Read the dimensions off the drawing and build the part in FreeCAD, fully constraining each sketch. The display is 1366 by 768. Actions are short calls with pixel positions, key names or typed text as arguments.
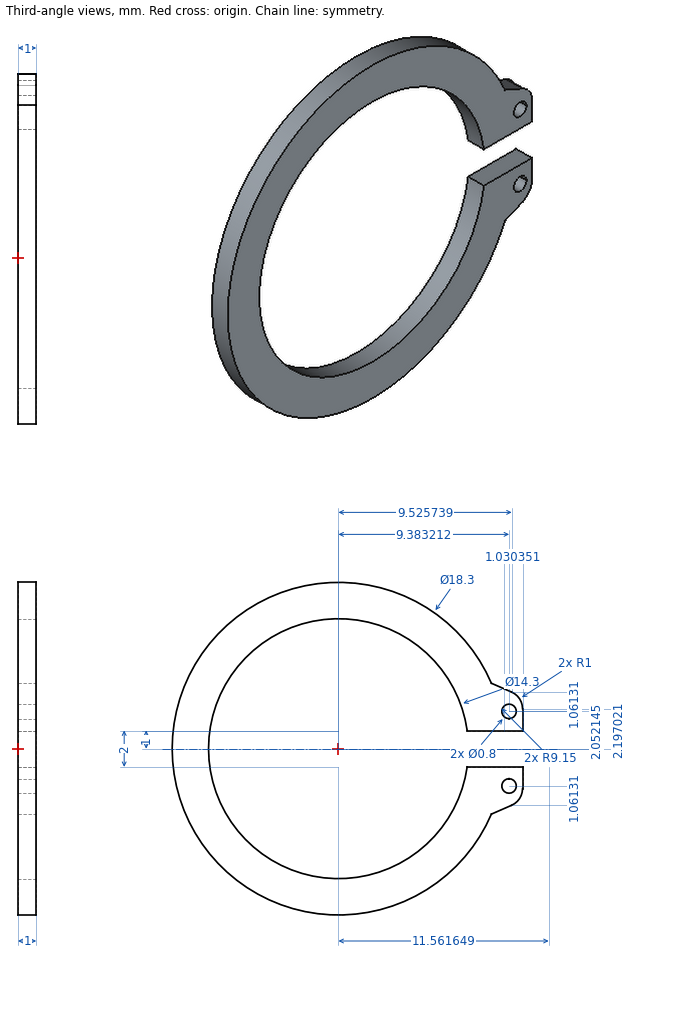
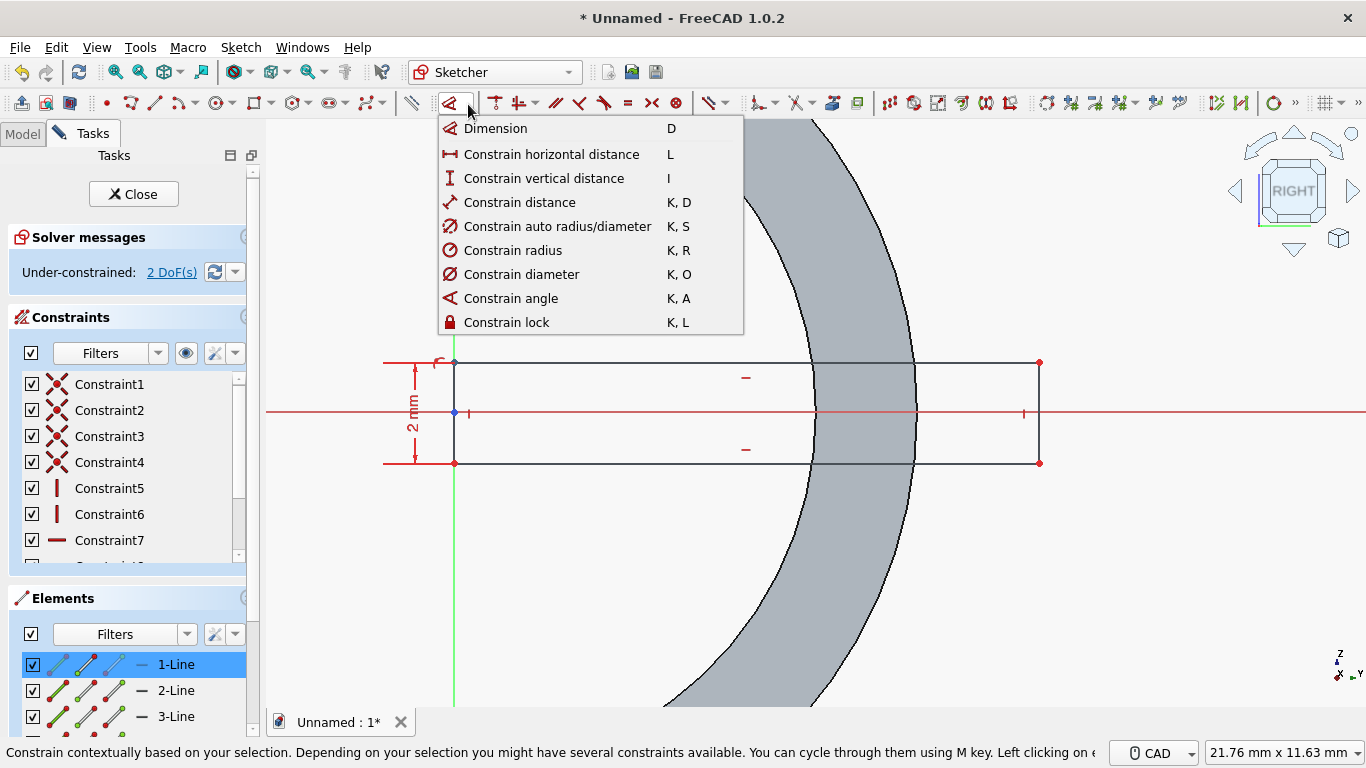
click(591, 178)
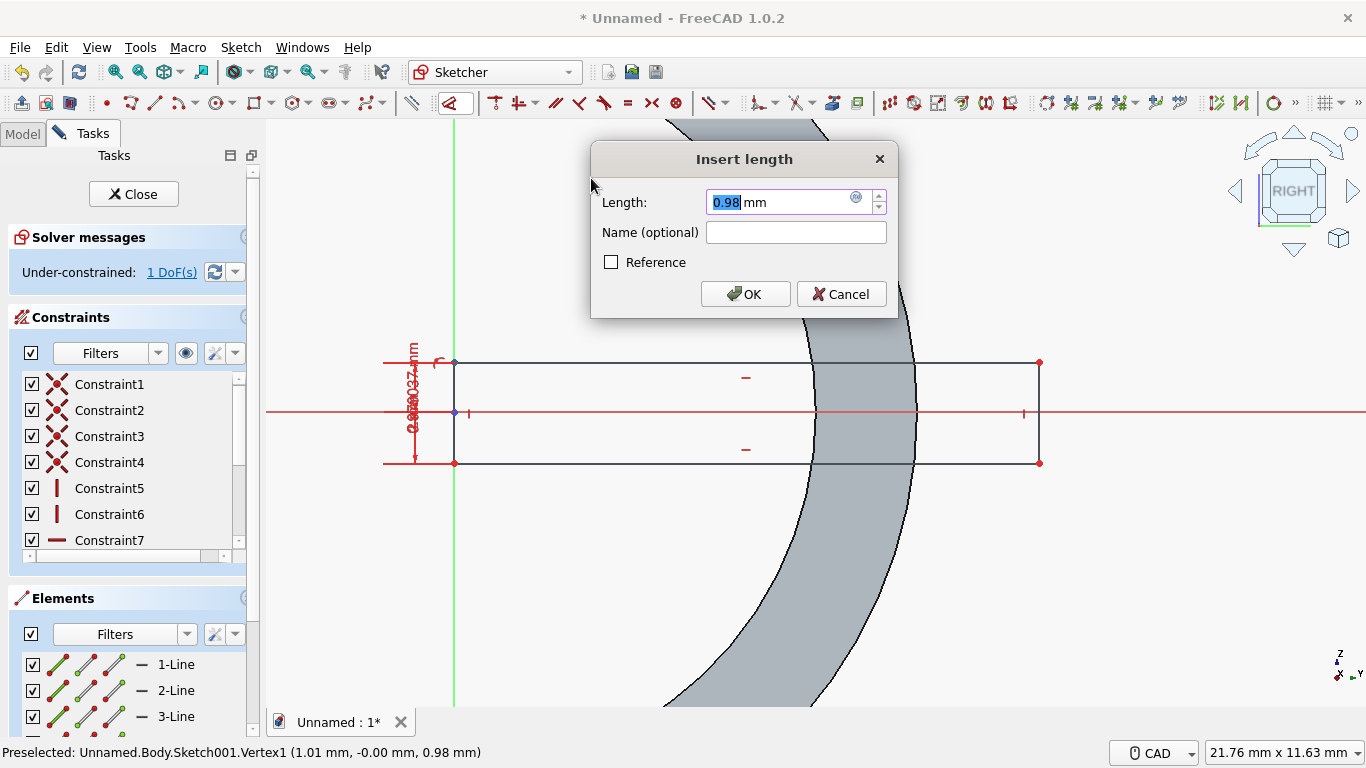
text(1)
key(Return)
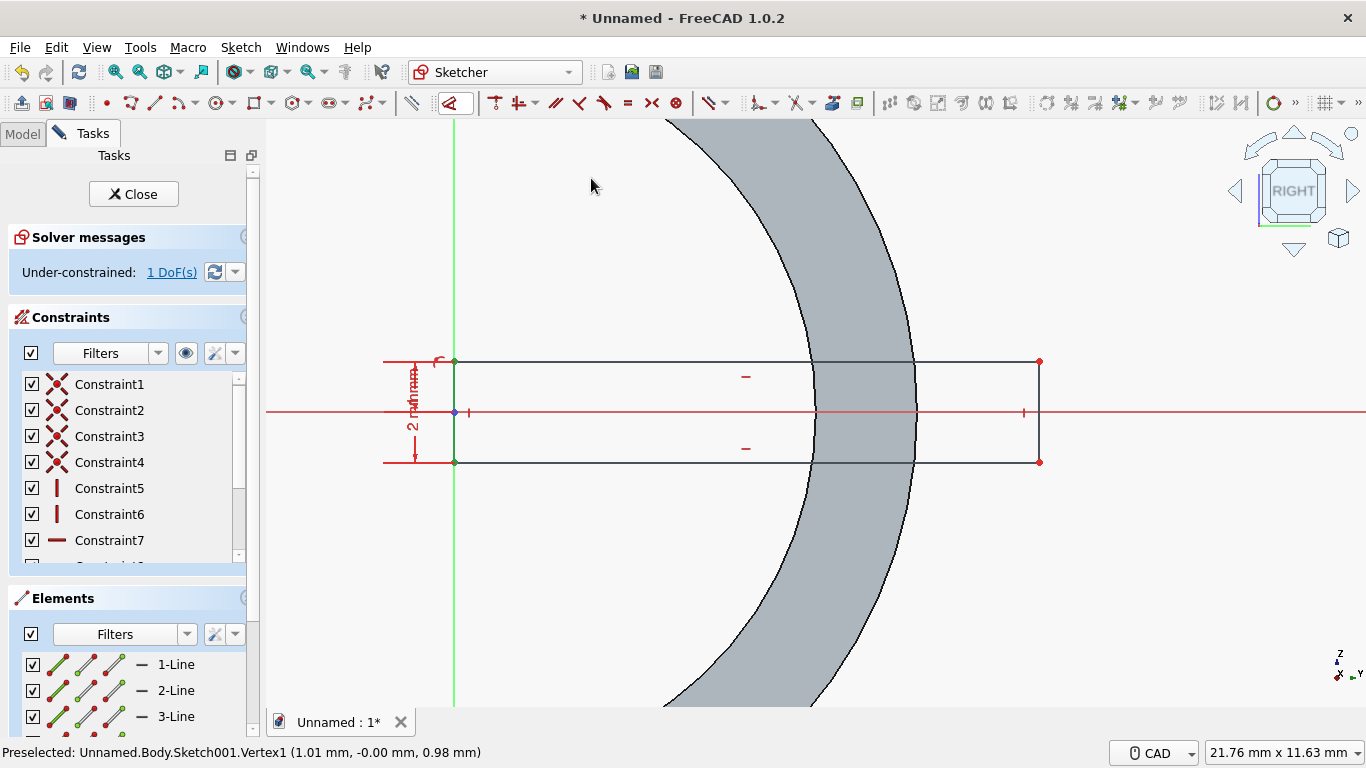
click(630, 463)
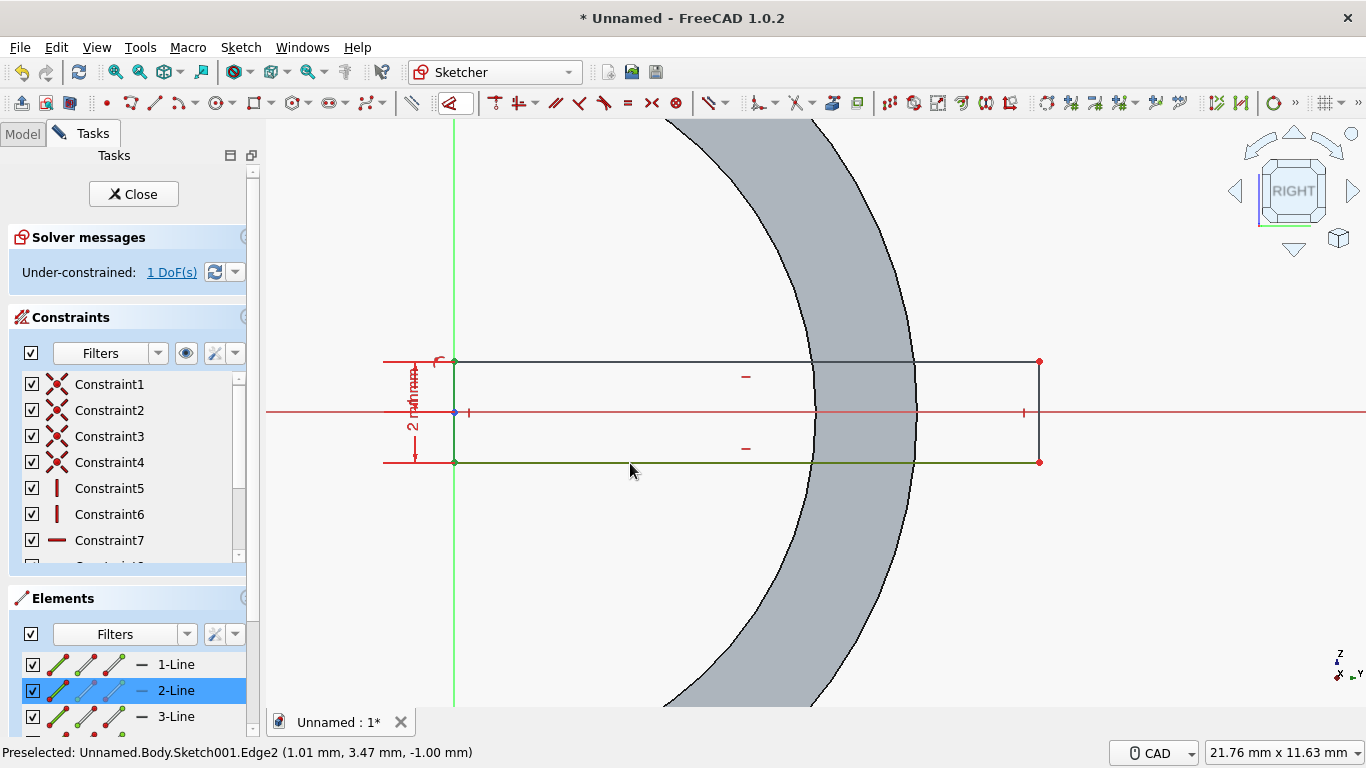
click(468, 104)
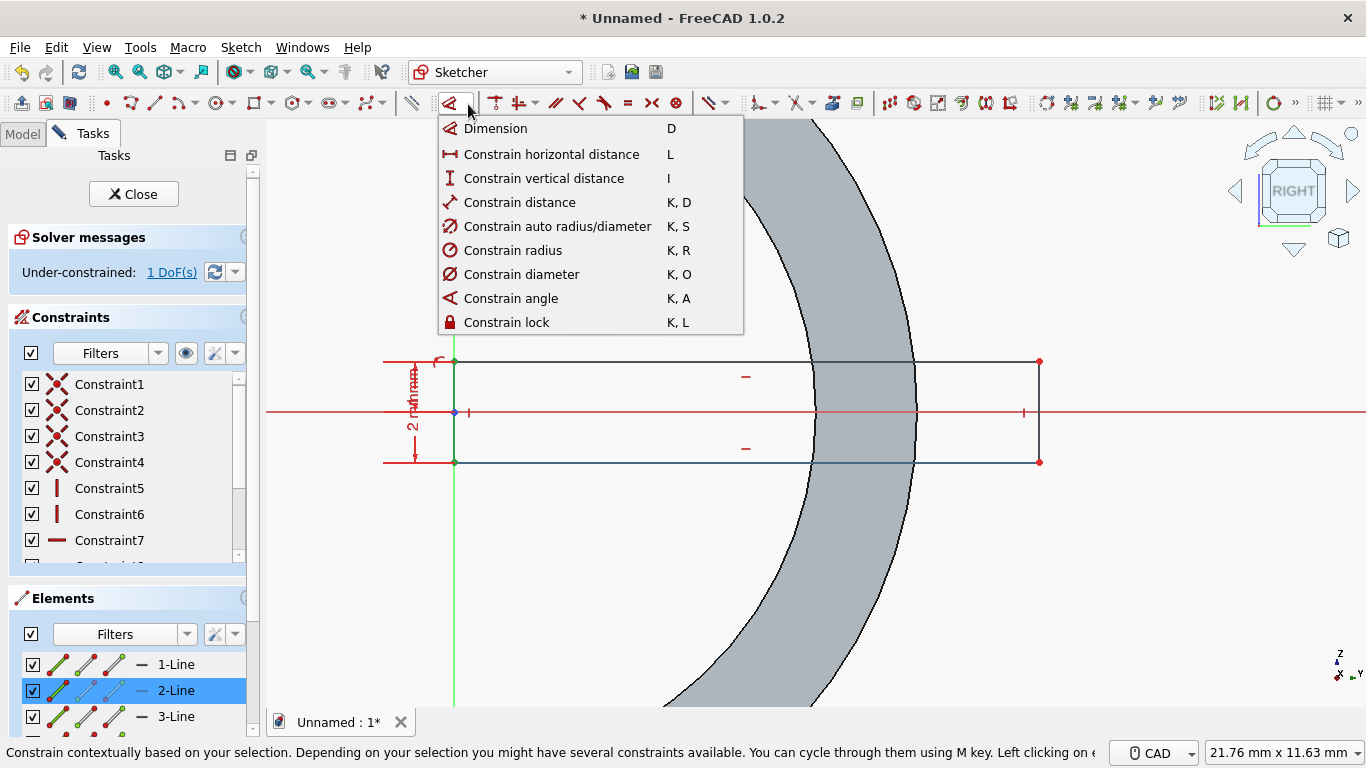
click(591, 154)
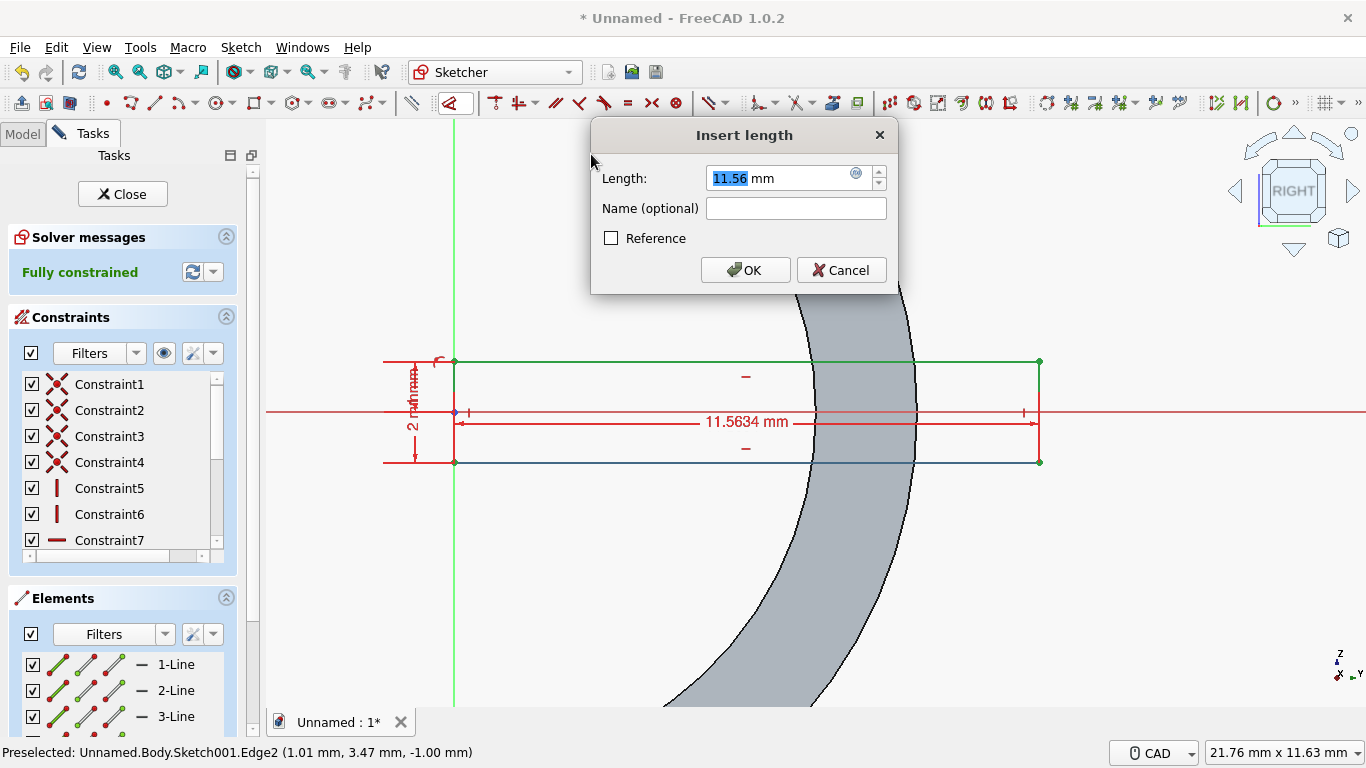
text(11.561649)
key(Return)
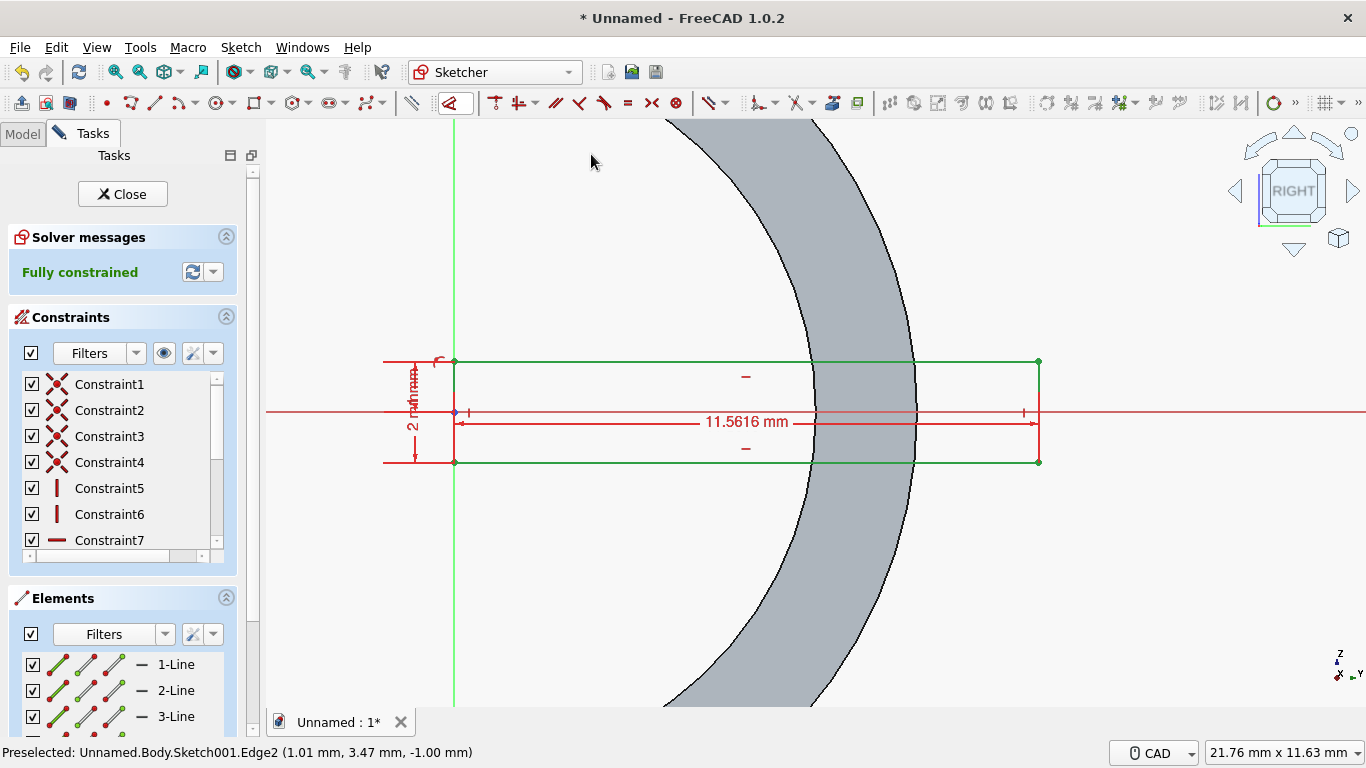
click(123, 194)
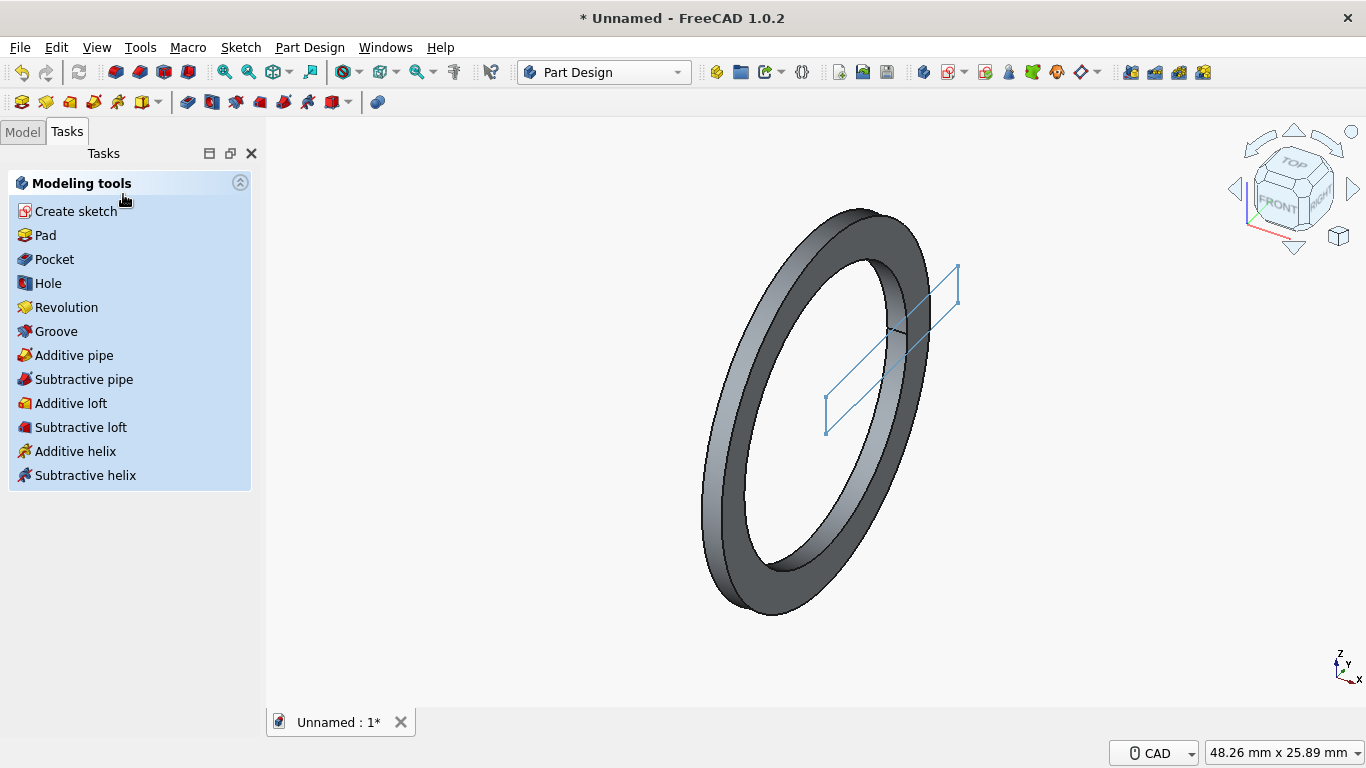
click(188, 102)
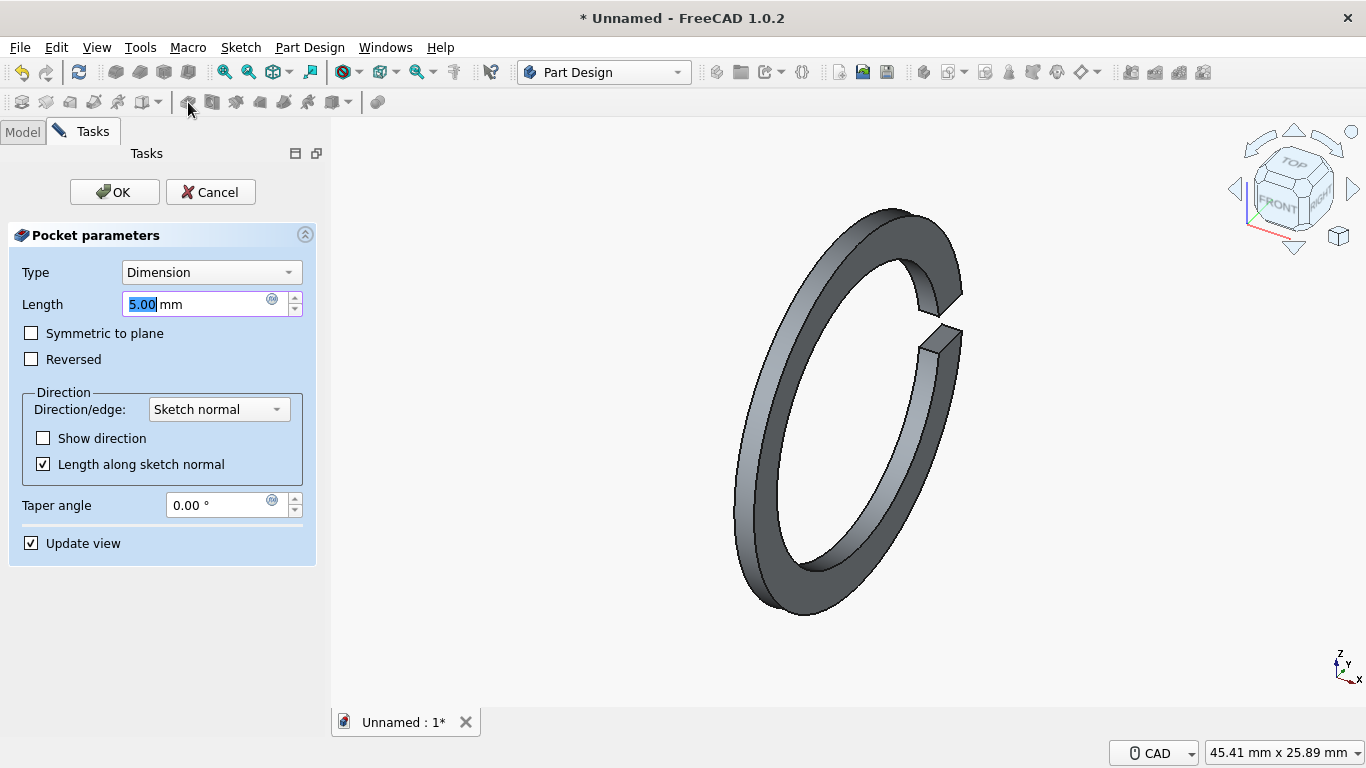
click(212, 272)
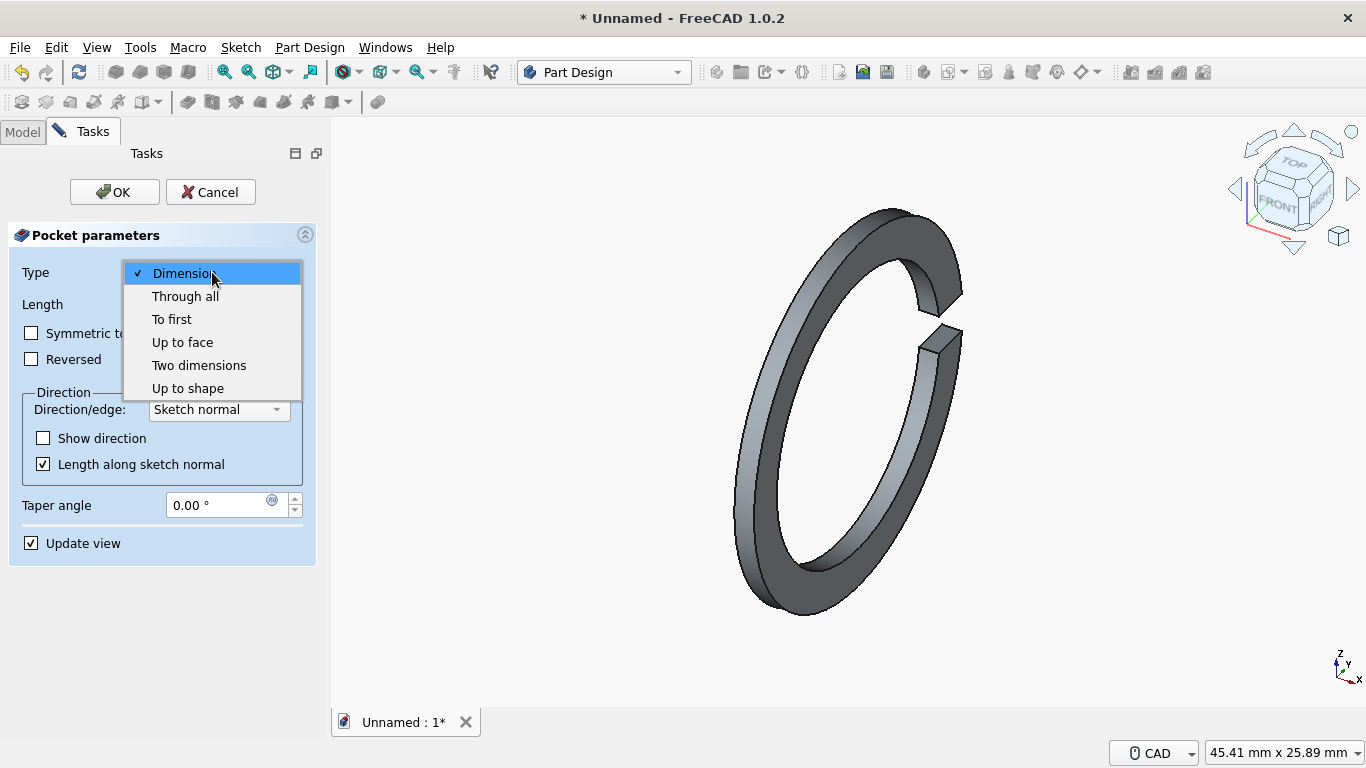
click(212, 296)